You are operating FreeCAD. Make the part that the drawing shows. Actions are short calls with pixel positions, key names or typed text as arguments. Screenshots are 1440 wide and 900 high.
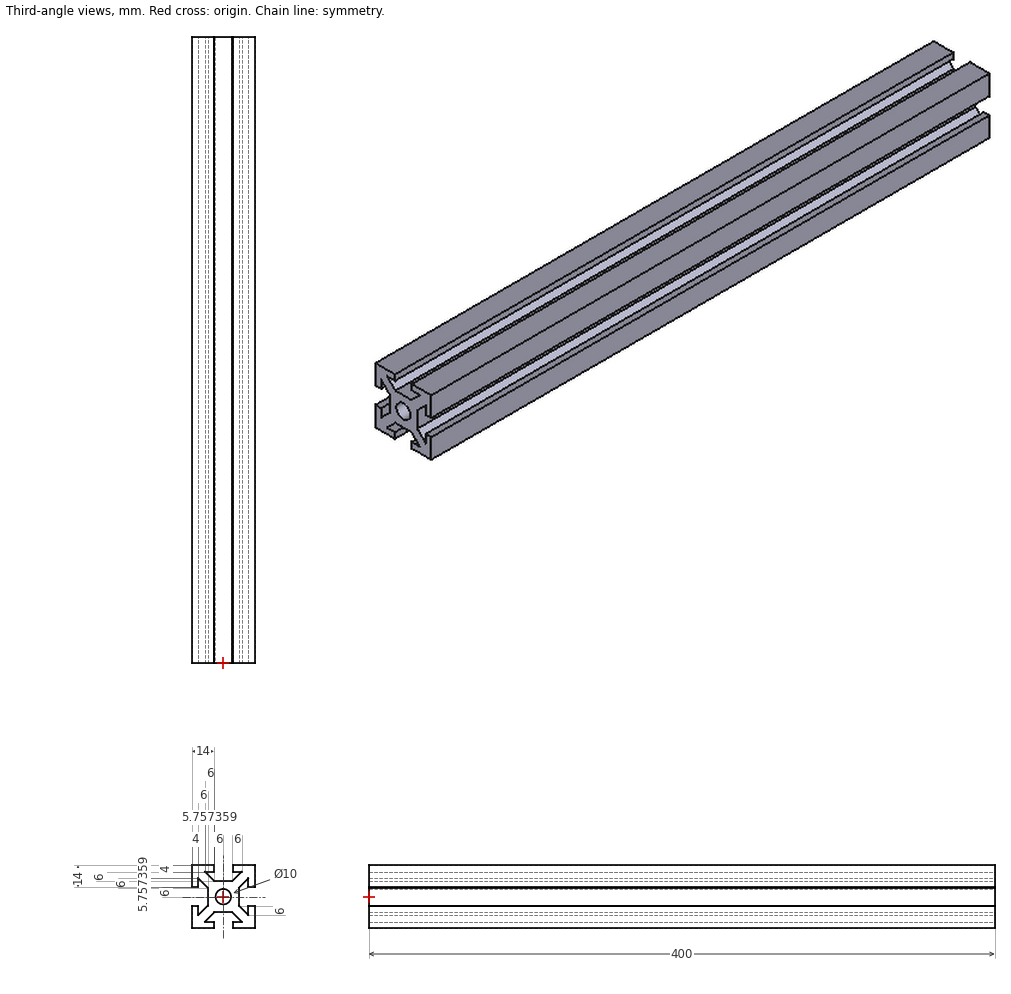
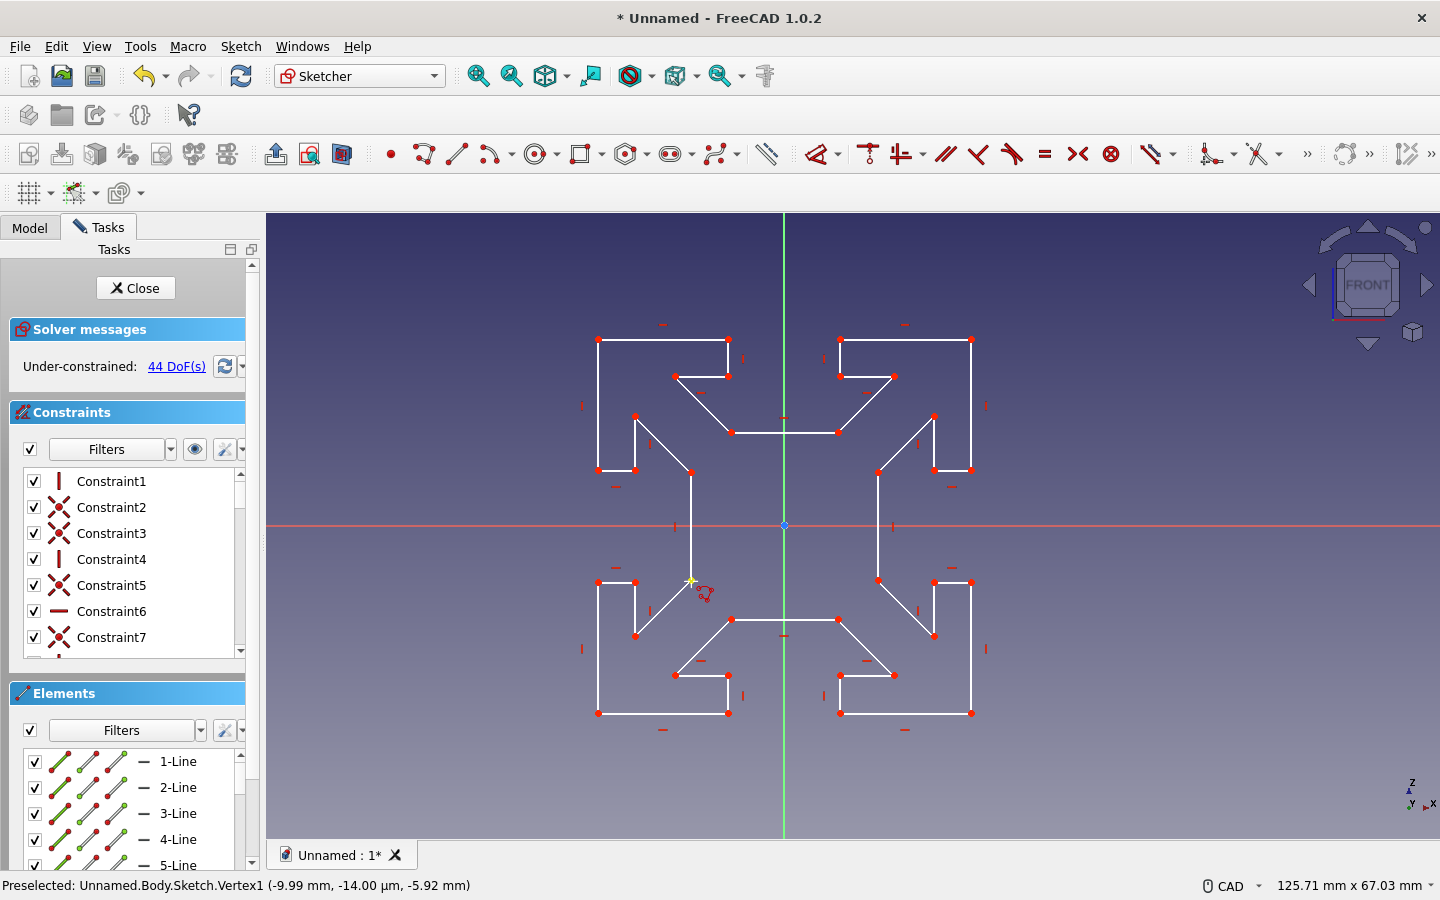
click(534, 154)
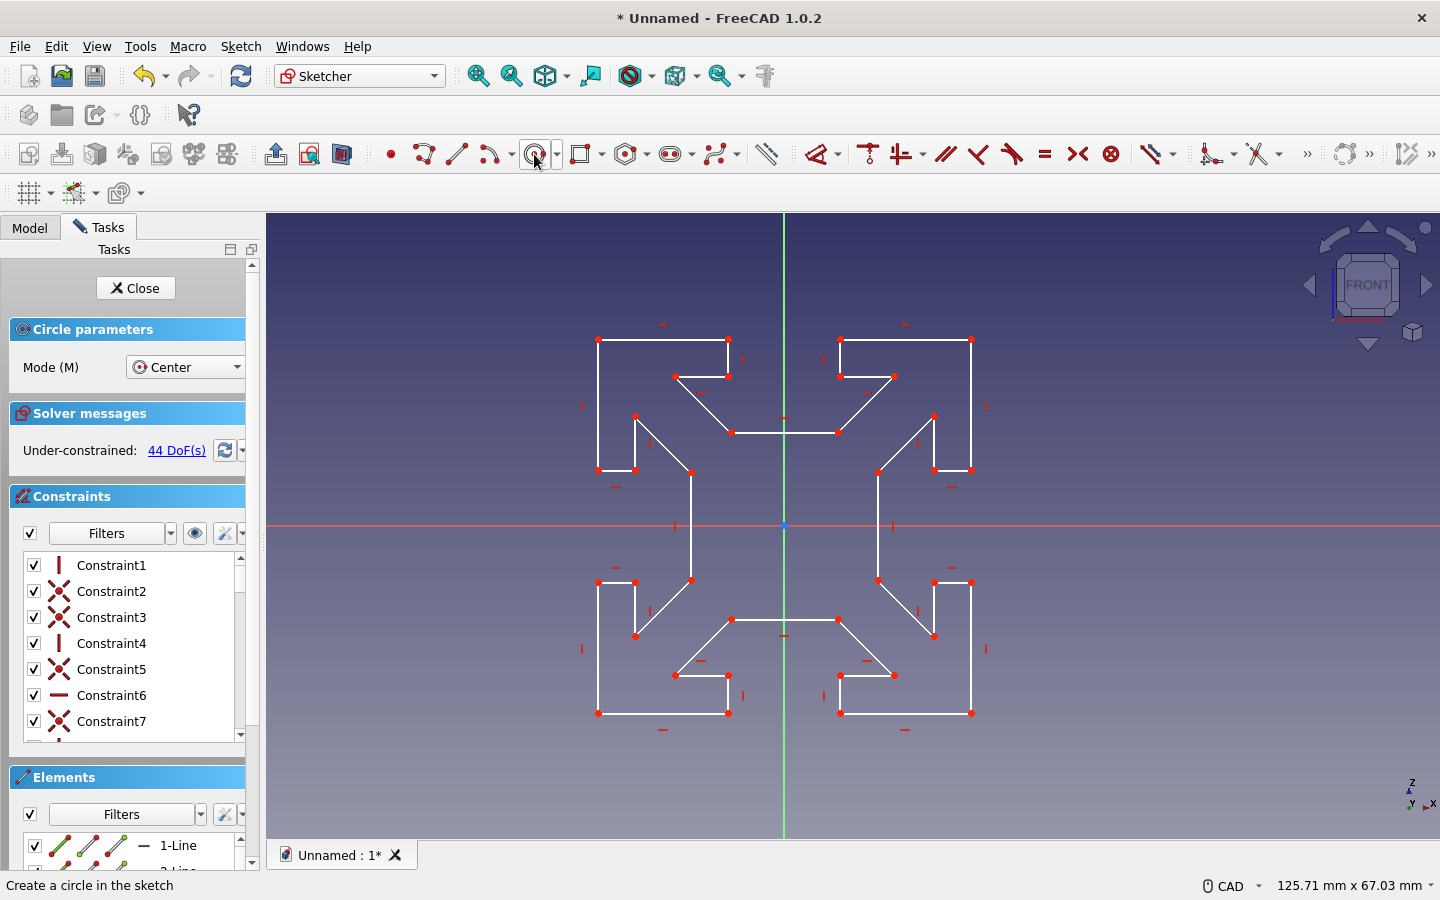
click(784, 526)
click(817, 493)
key(Escape)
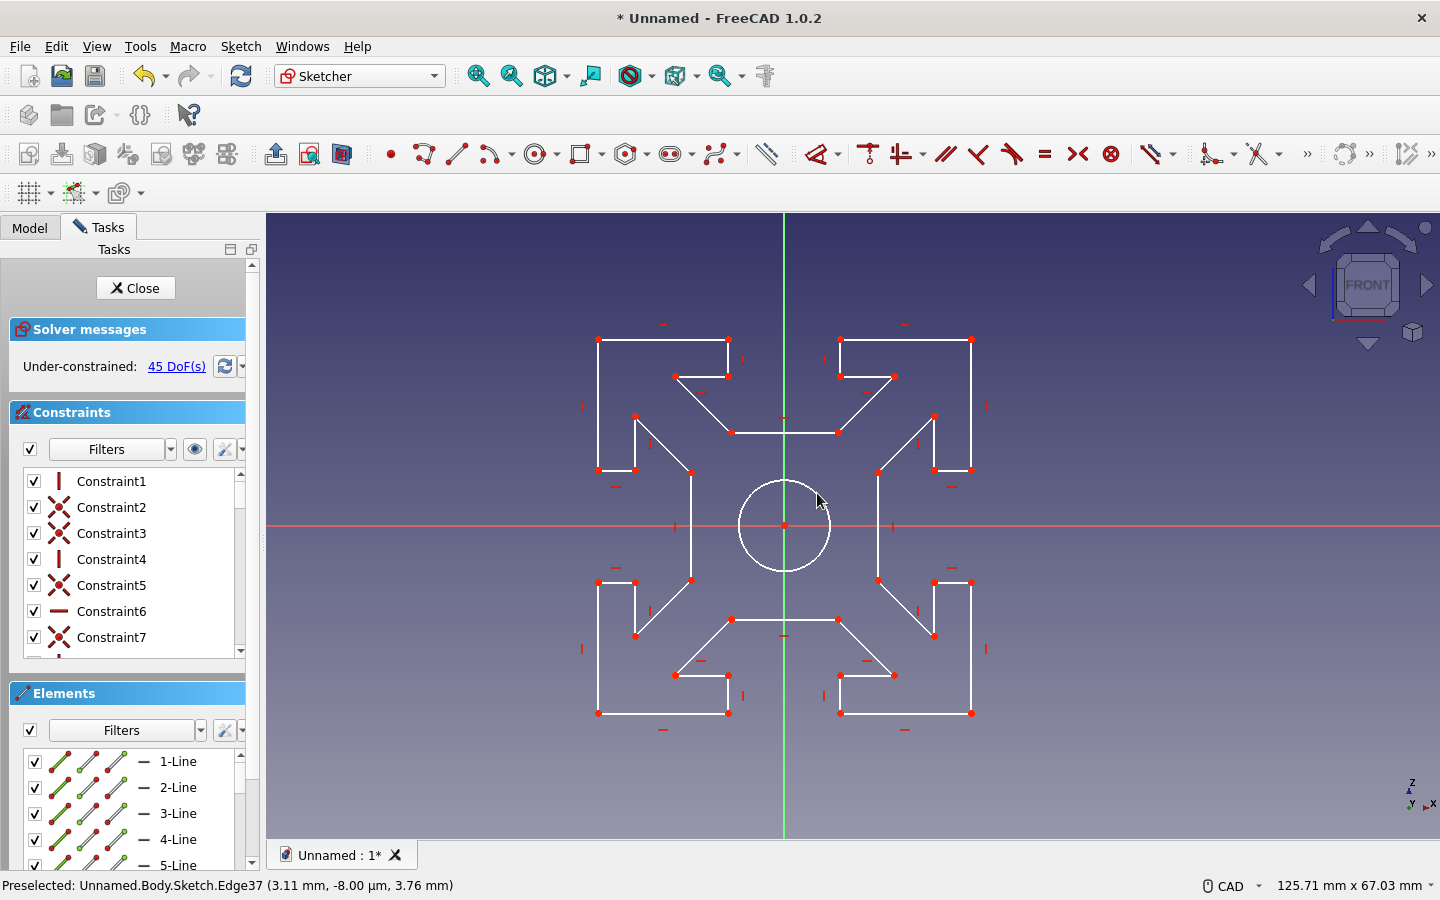
click(675, 377)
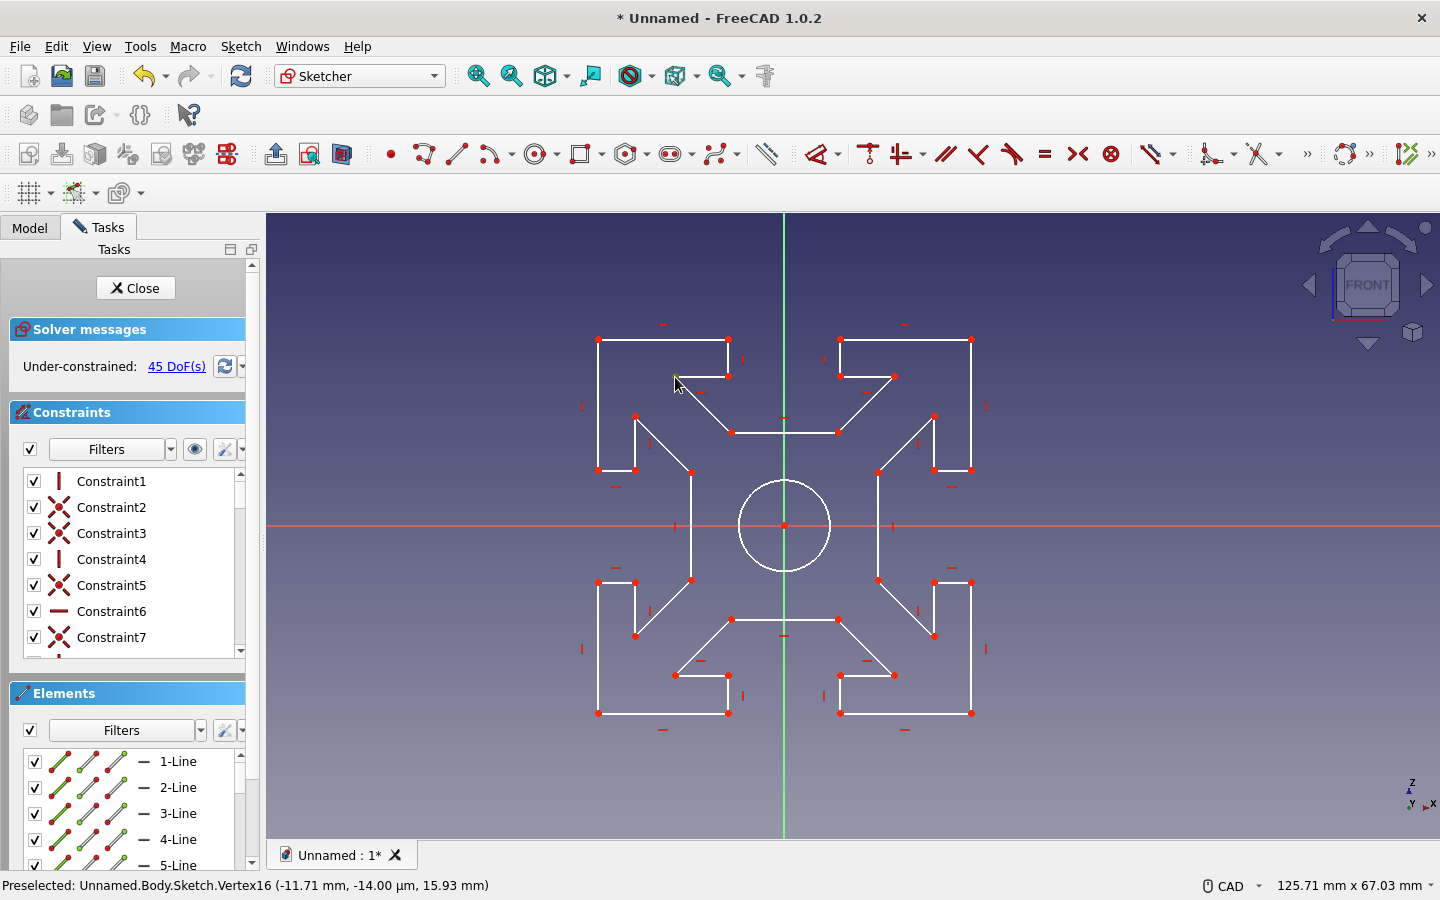
click(894, 377)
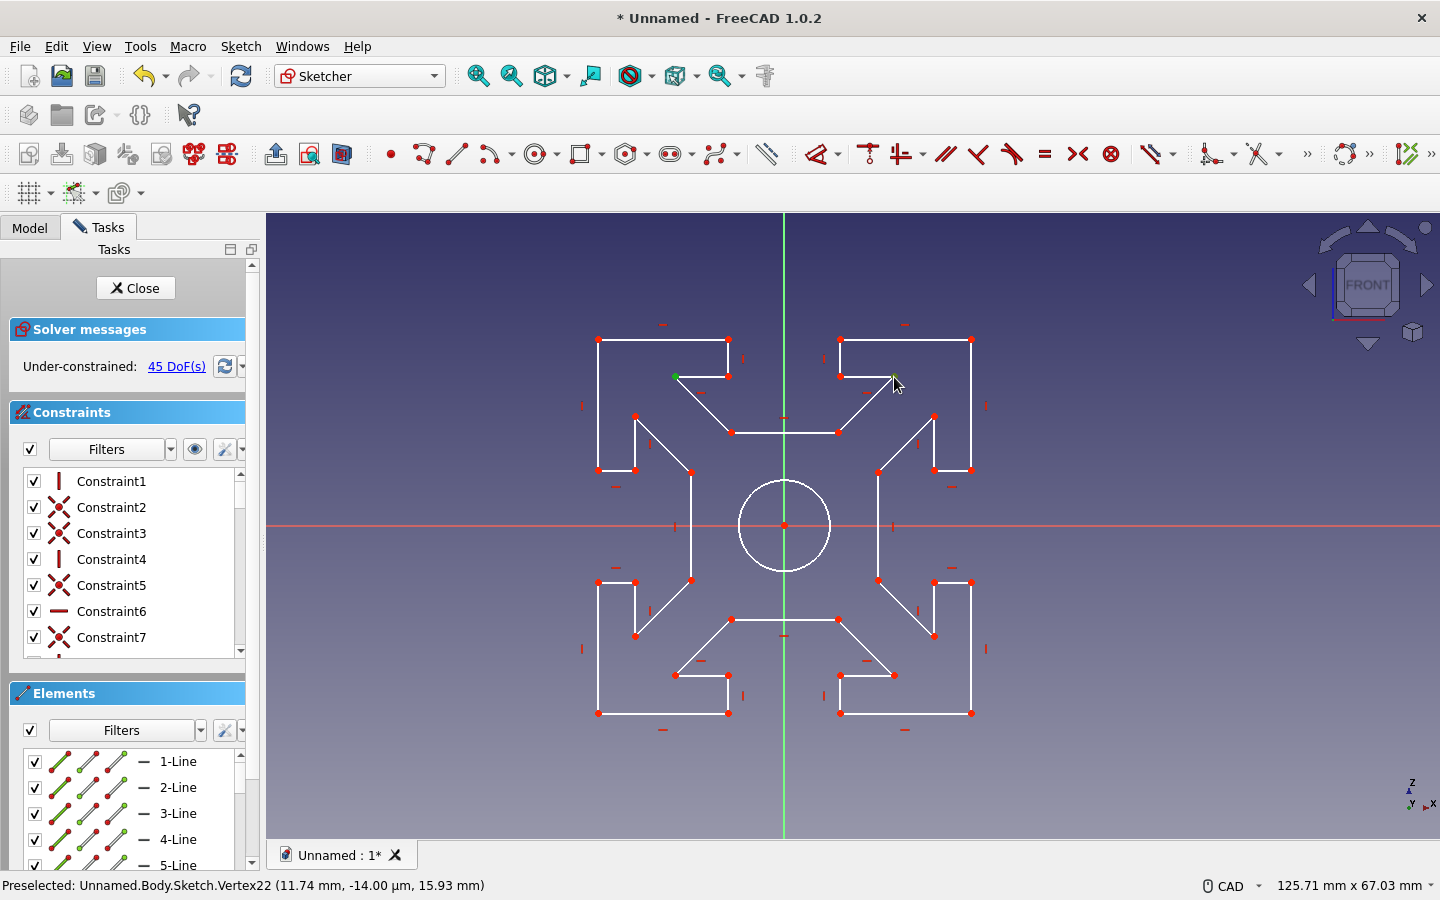
click(784, 770)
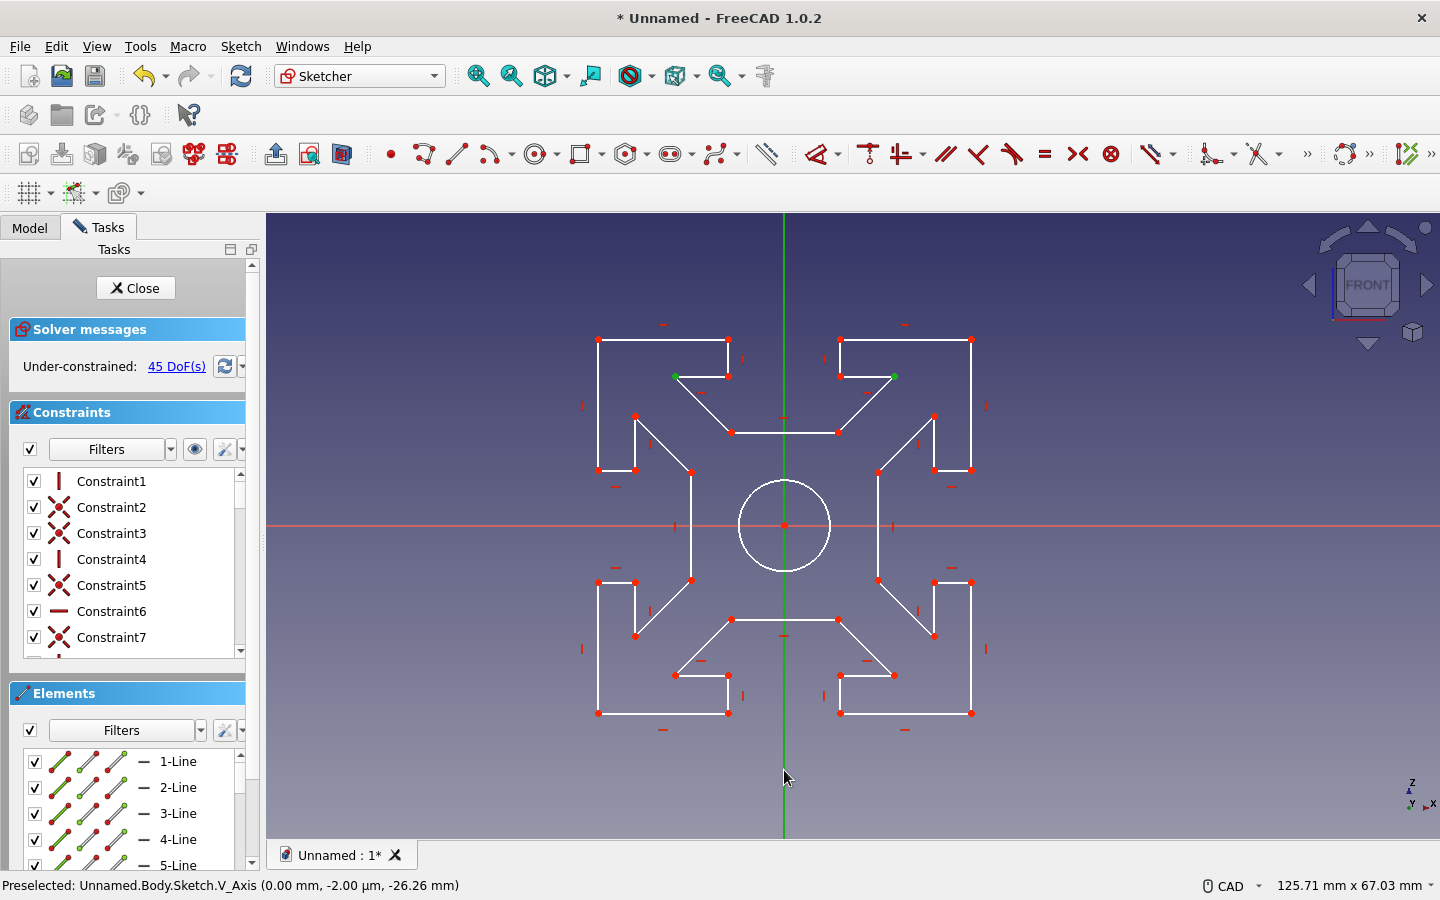
key(s)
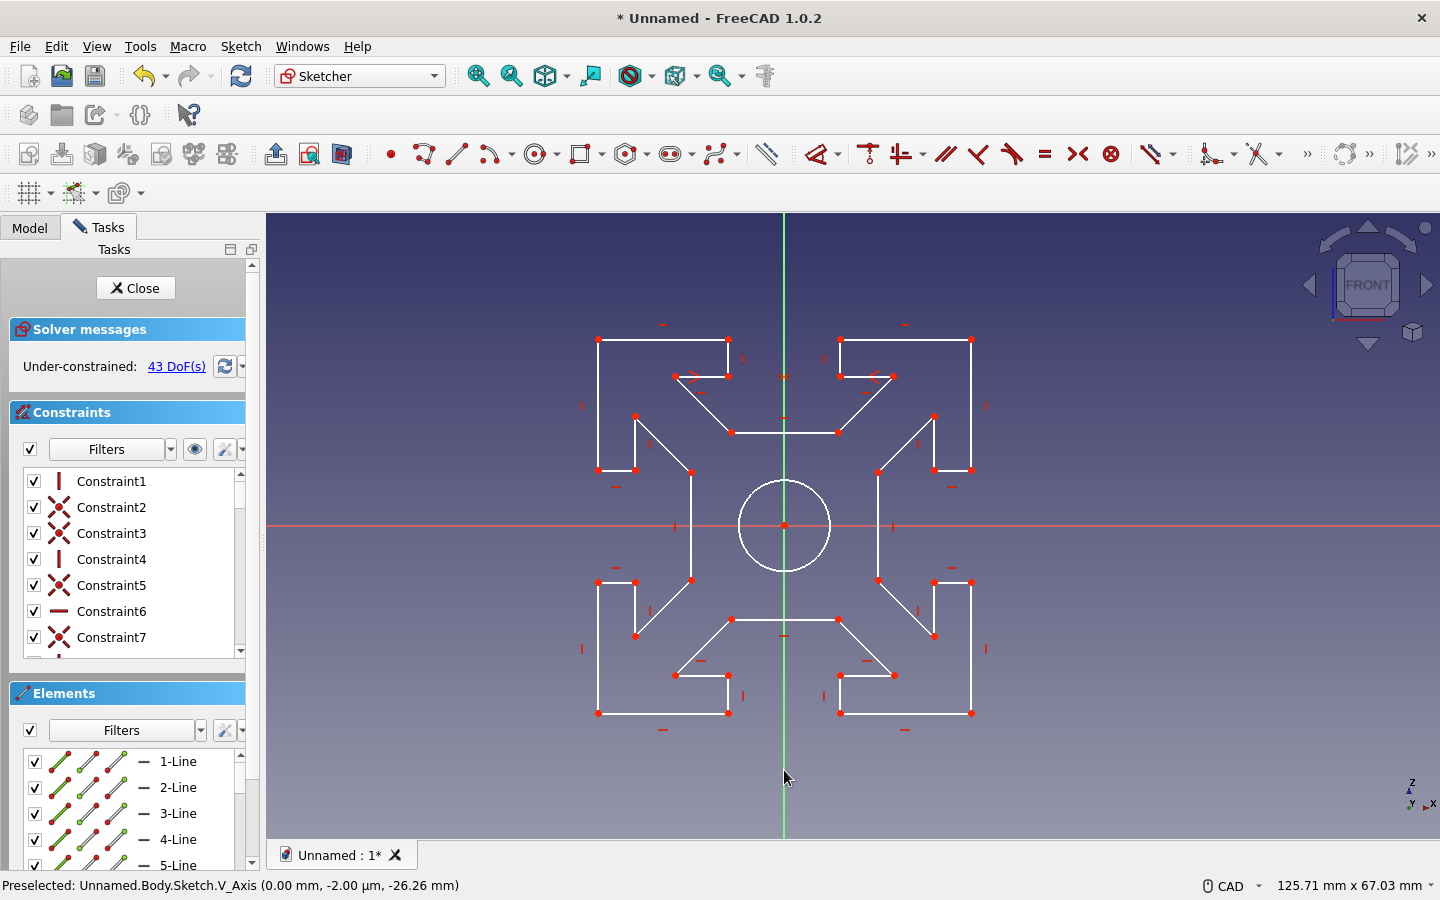
click(728, 340)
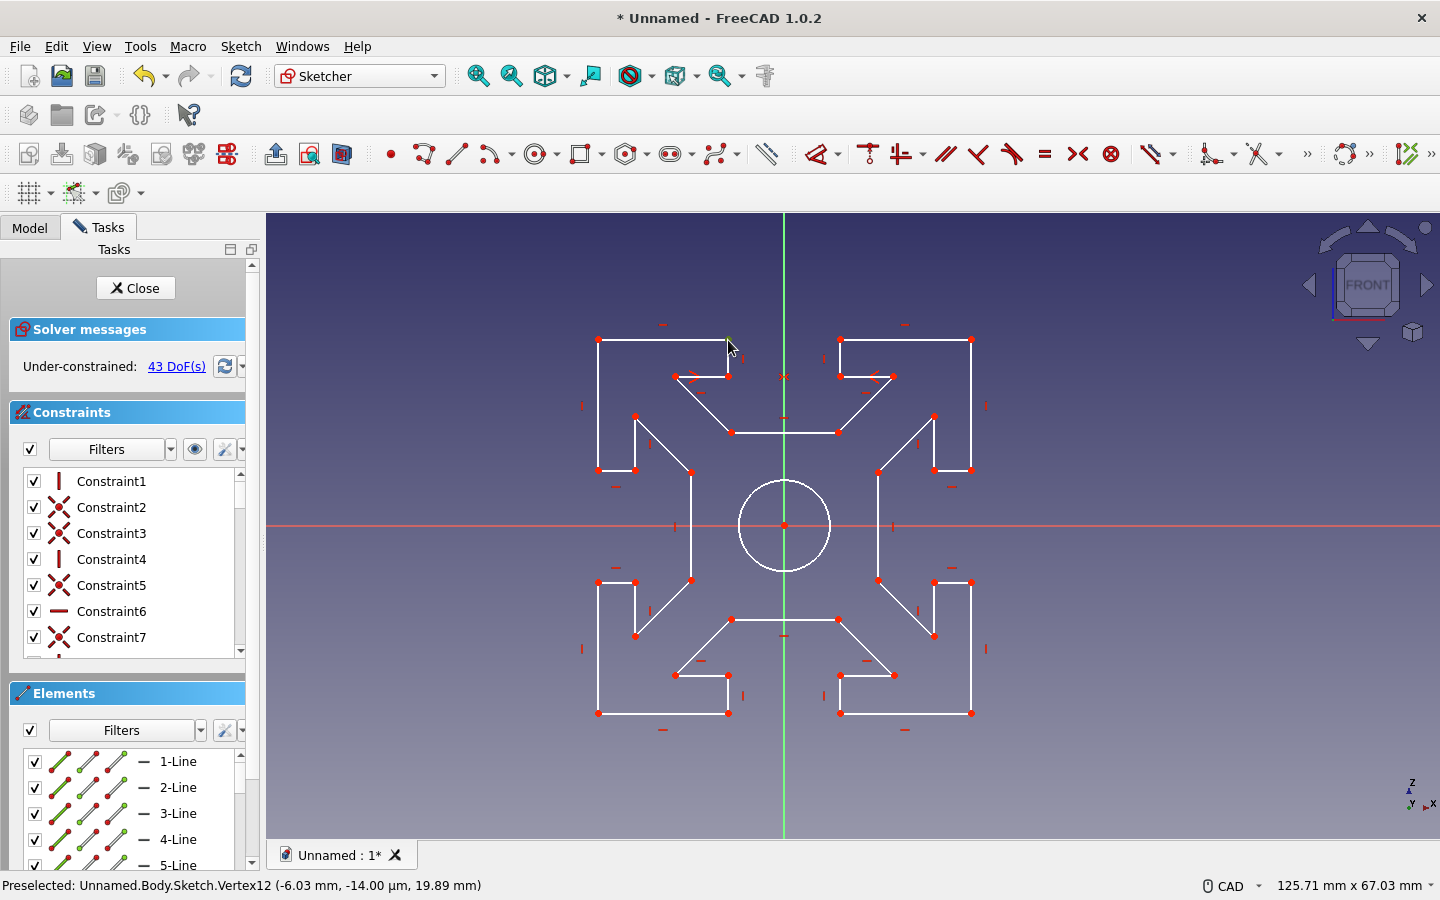
click(840, 340)